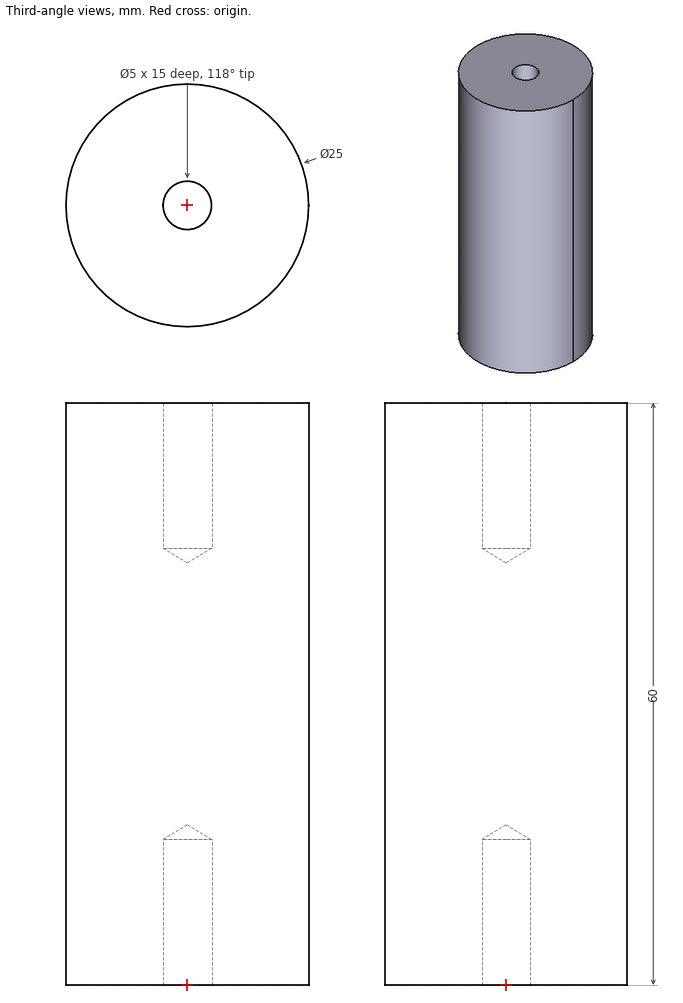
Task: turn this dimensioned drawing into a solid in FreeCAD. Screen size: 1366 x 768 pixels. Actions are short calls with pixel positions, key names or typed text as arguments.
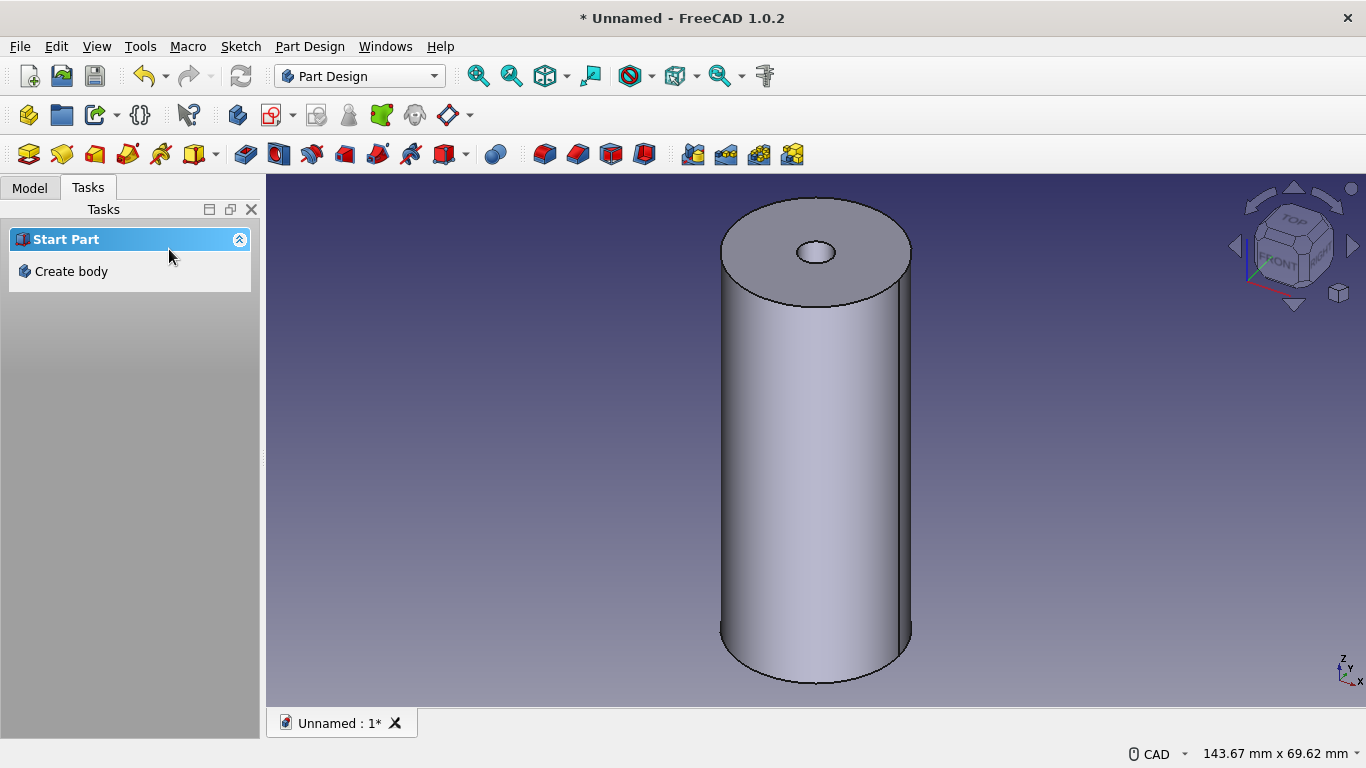
key(5)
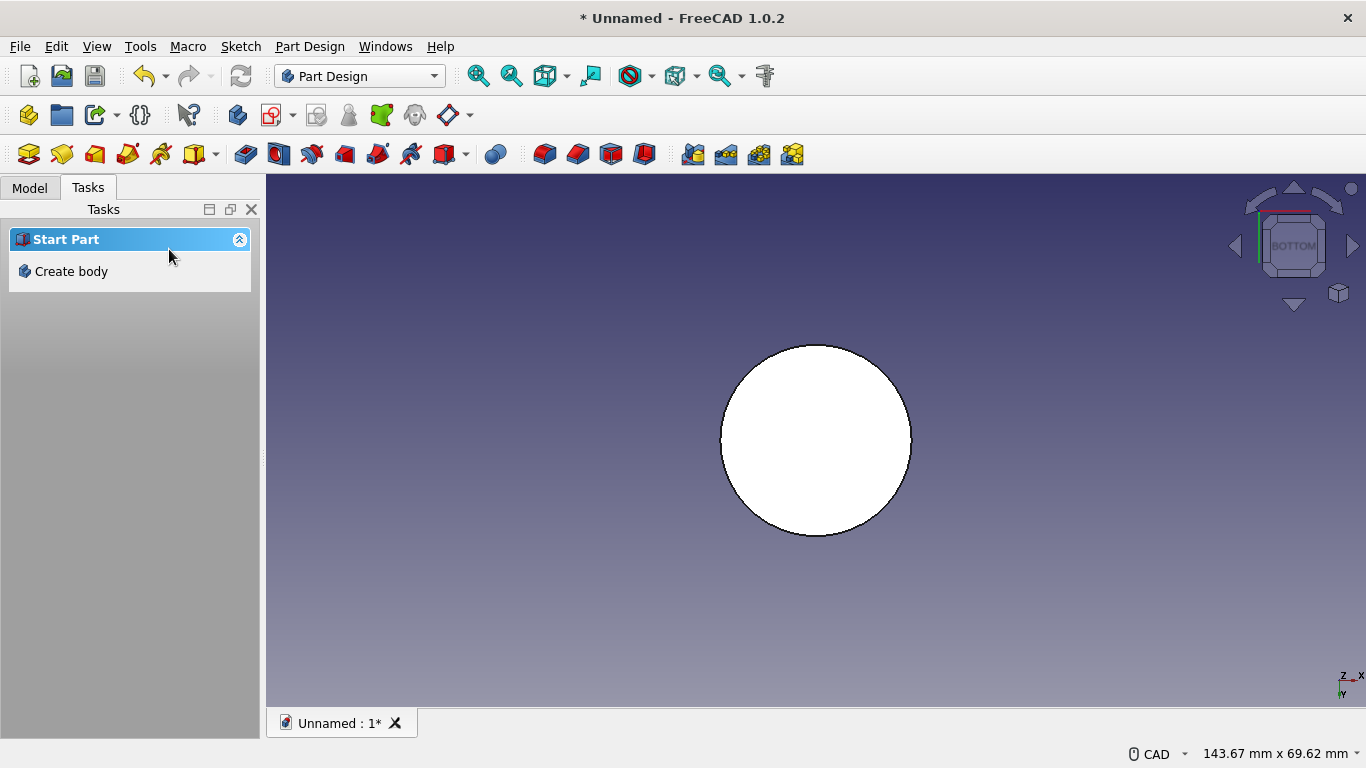
click(479, 76)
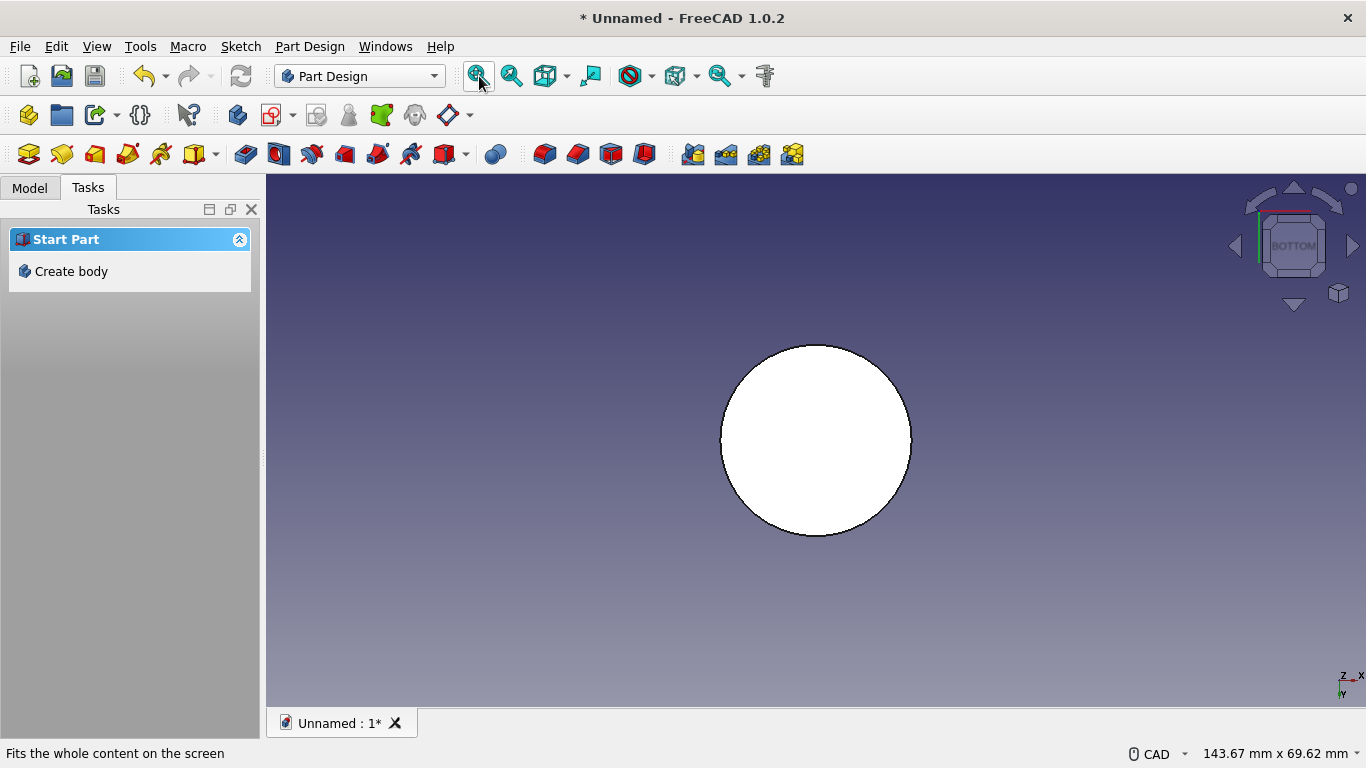
click(816, 439)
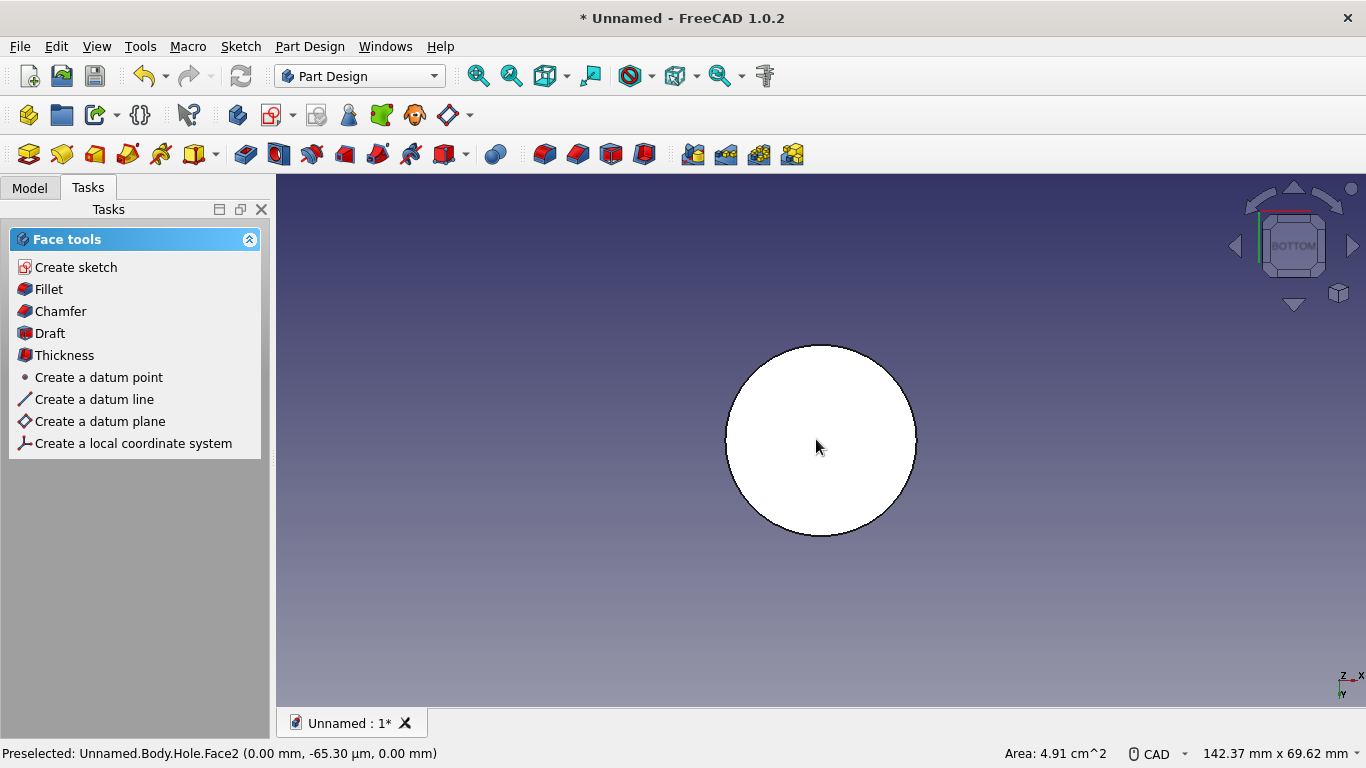
click(270, 116)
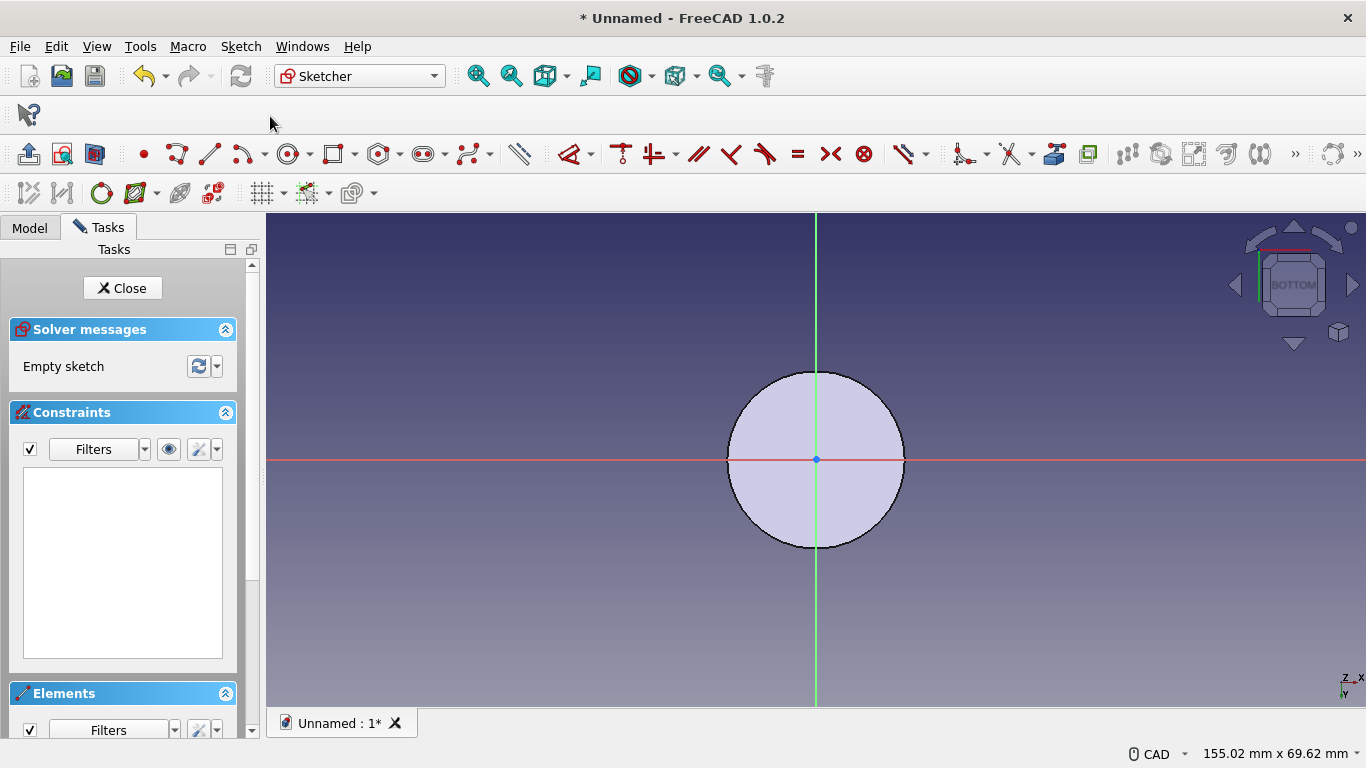
scroll(825, 460, up, 11)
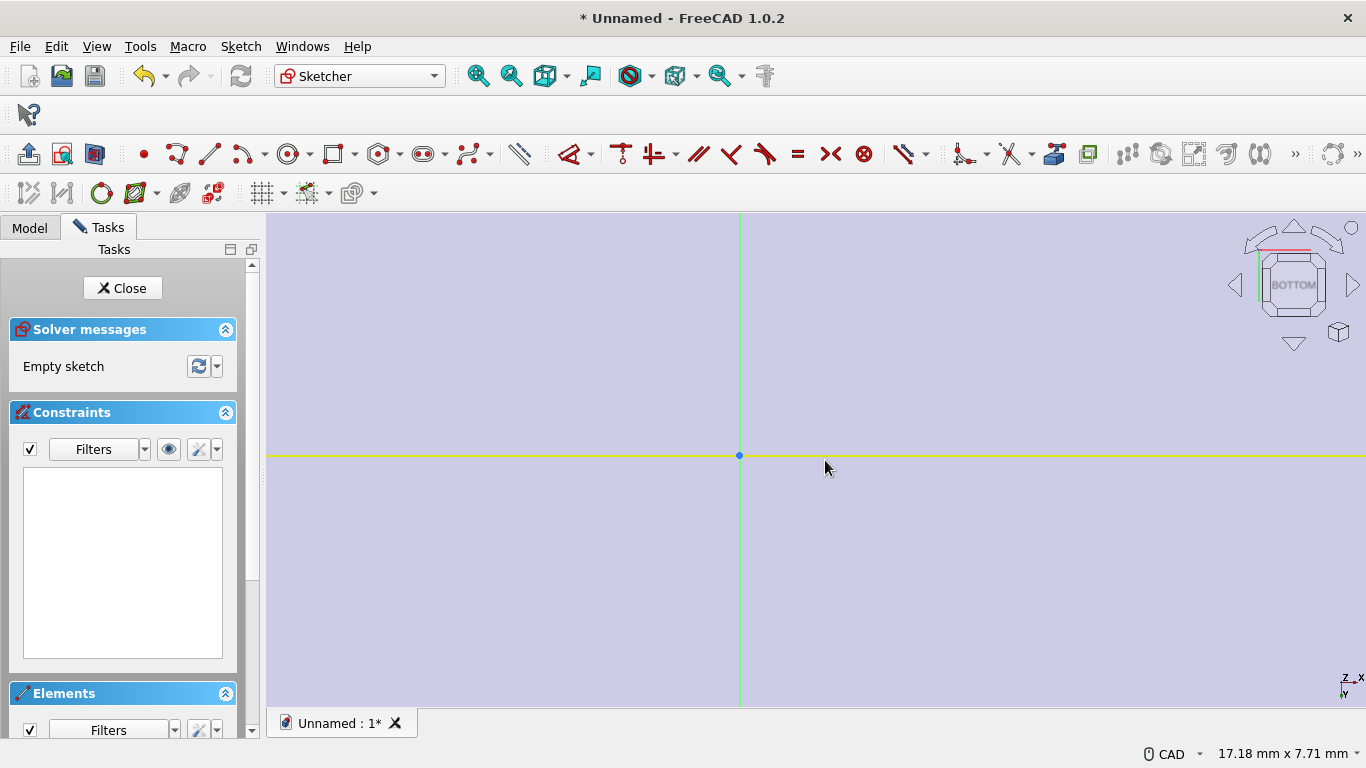
click(288, 154)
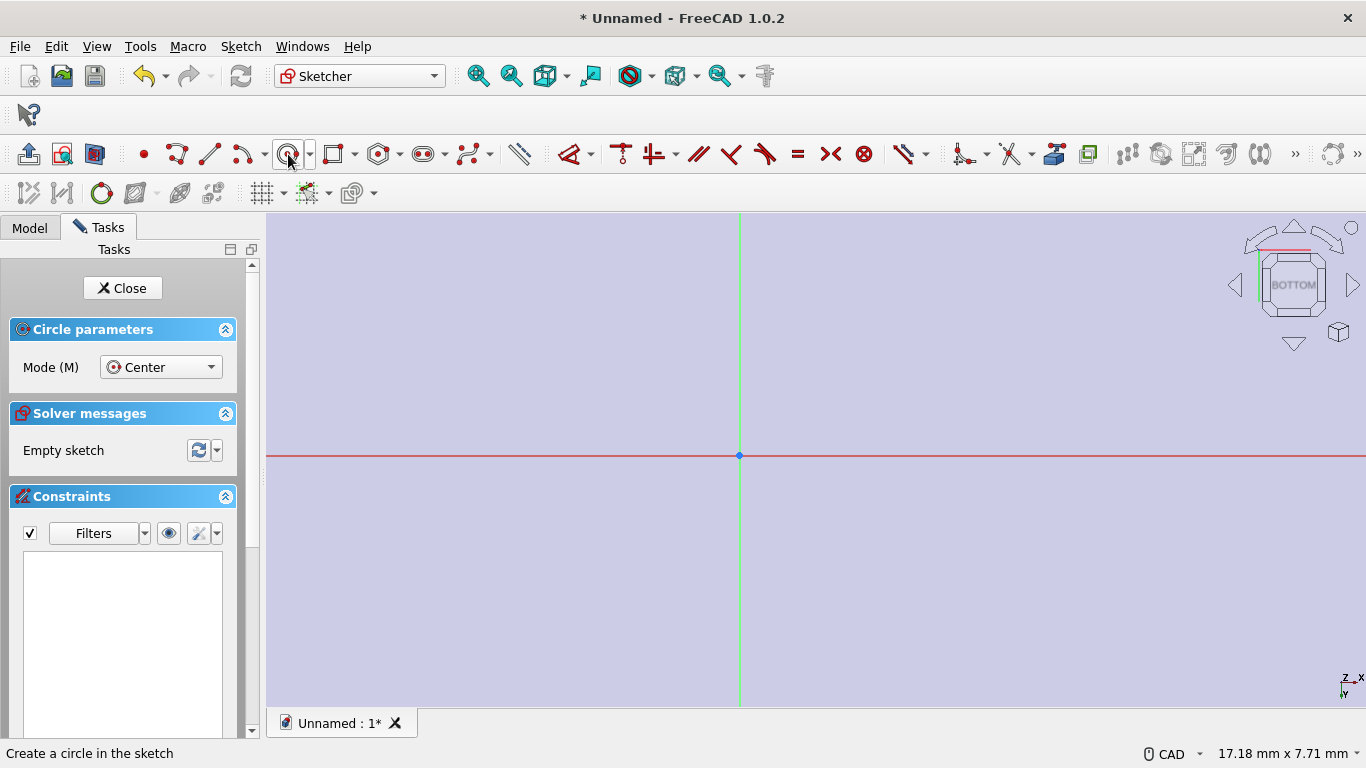
click(740, 456)
click(853, 343)
key(Escape)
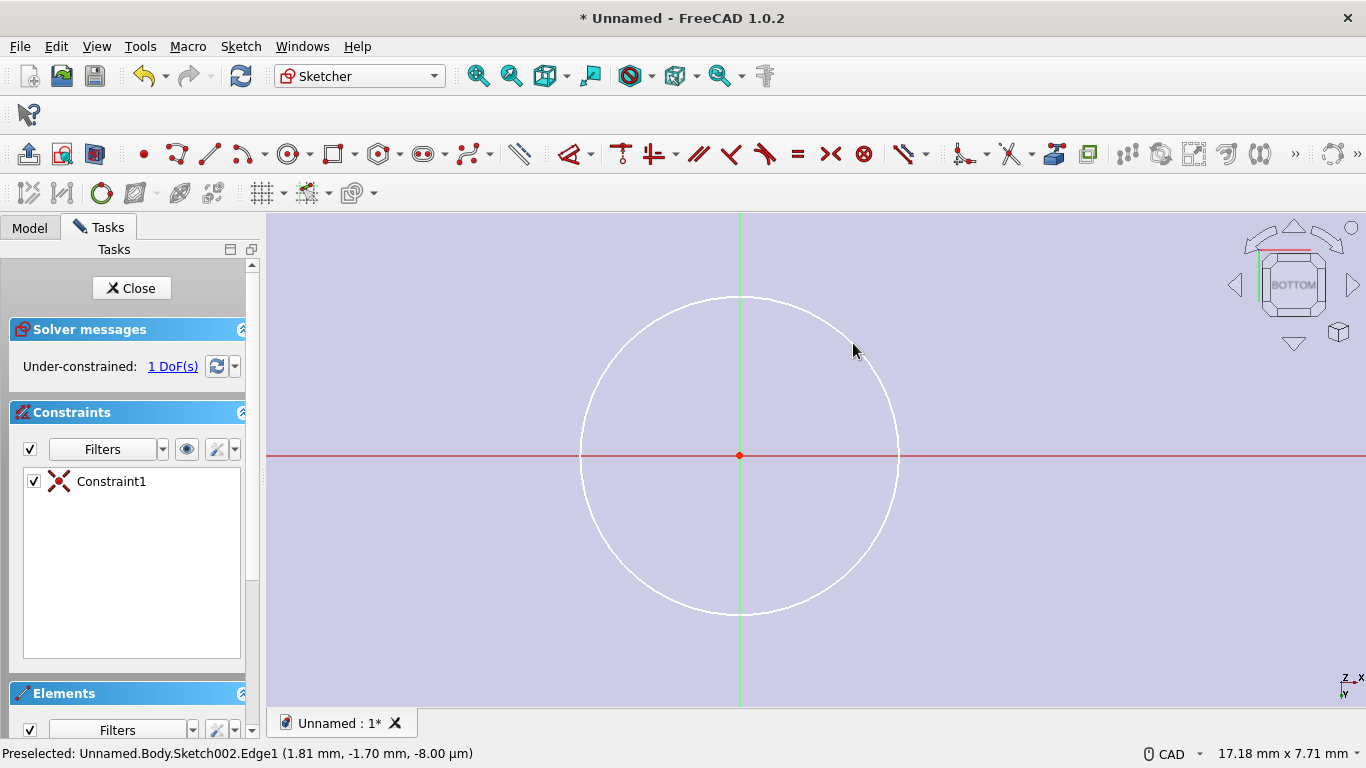
click(568, 154)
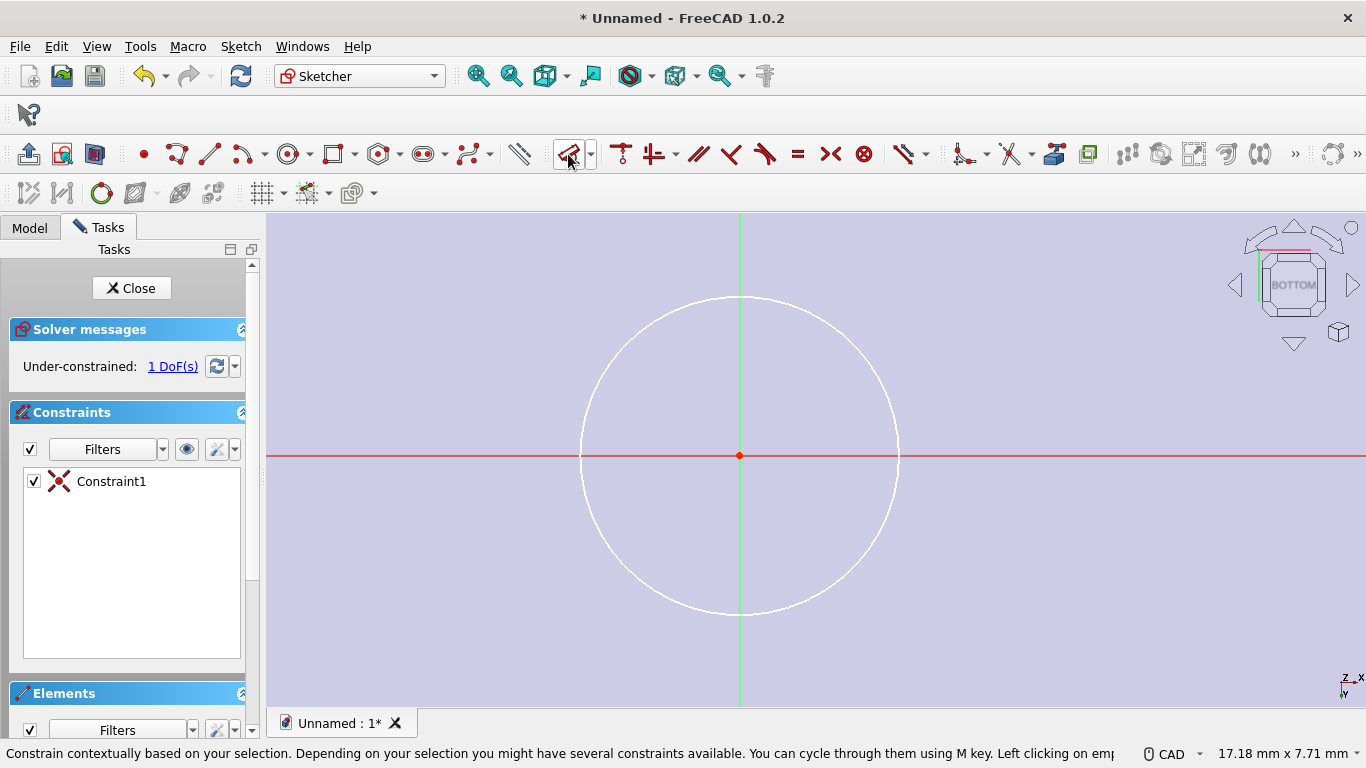
click(852, 343)
click(875, 320)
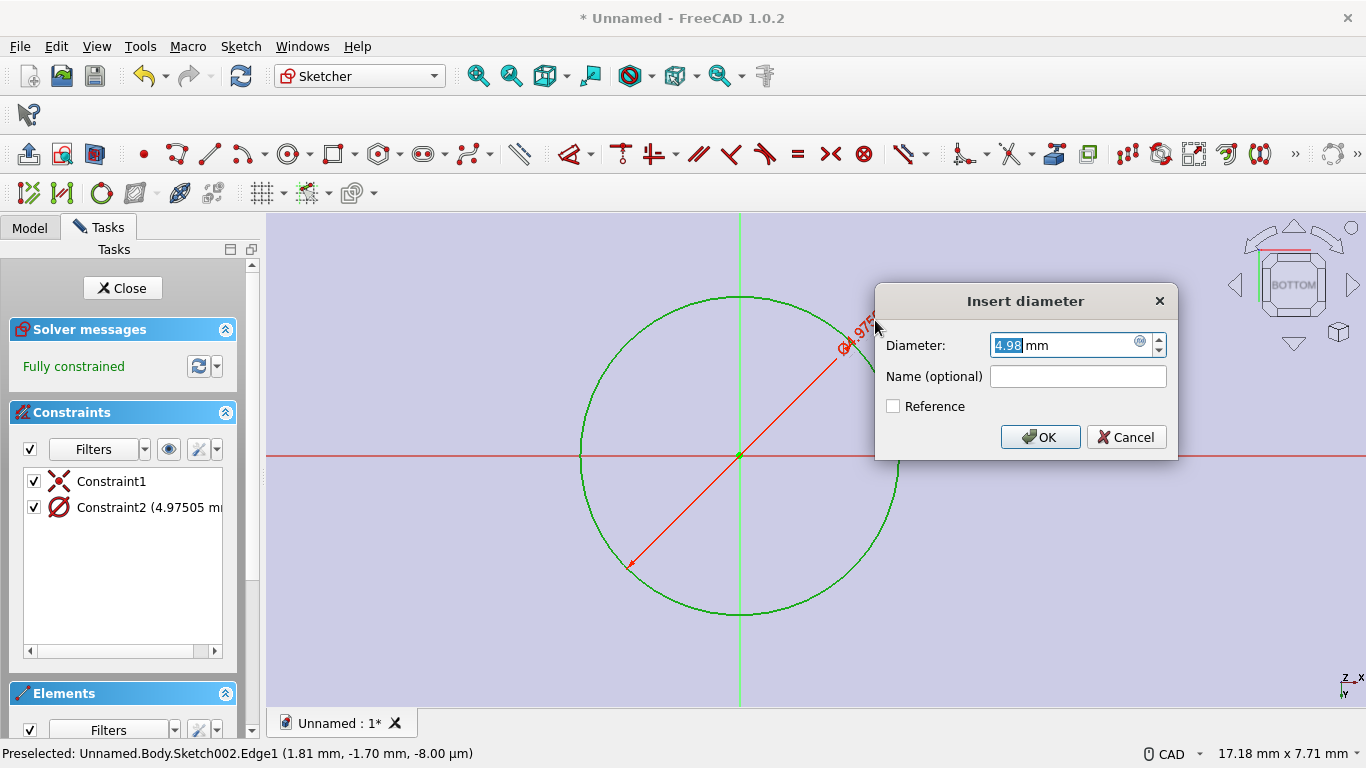
text(5)
key(Return)
key(Escape)